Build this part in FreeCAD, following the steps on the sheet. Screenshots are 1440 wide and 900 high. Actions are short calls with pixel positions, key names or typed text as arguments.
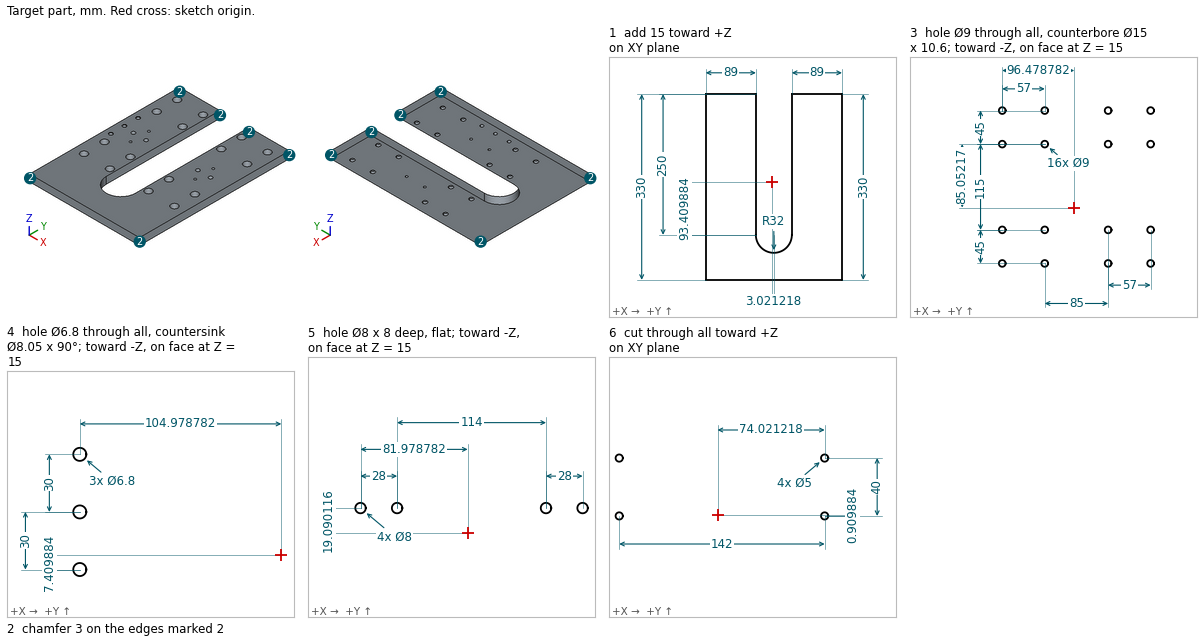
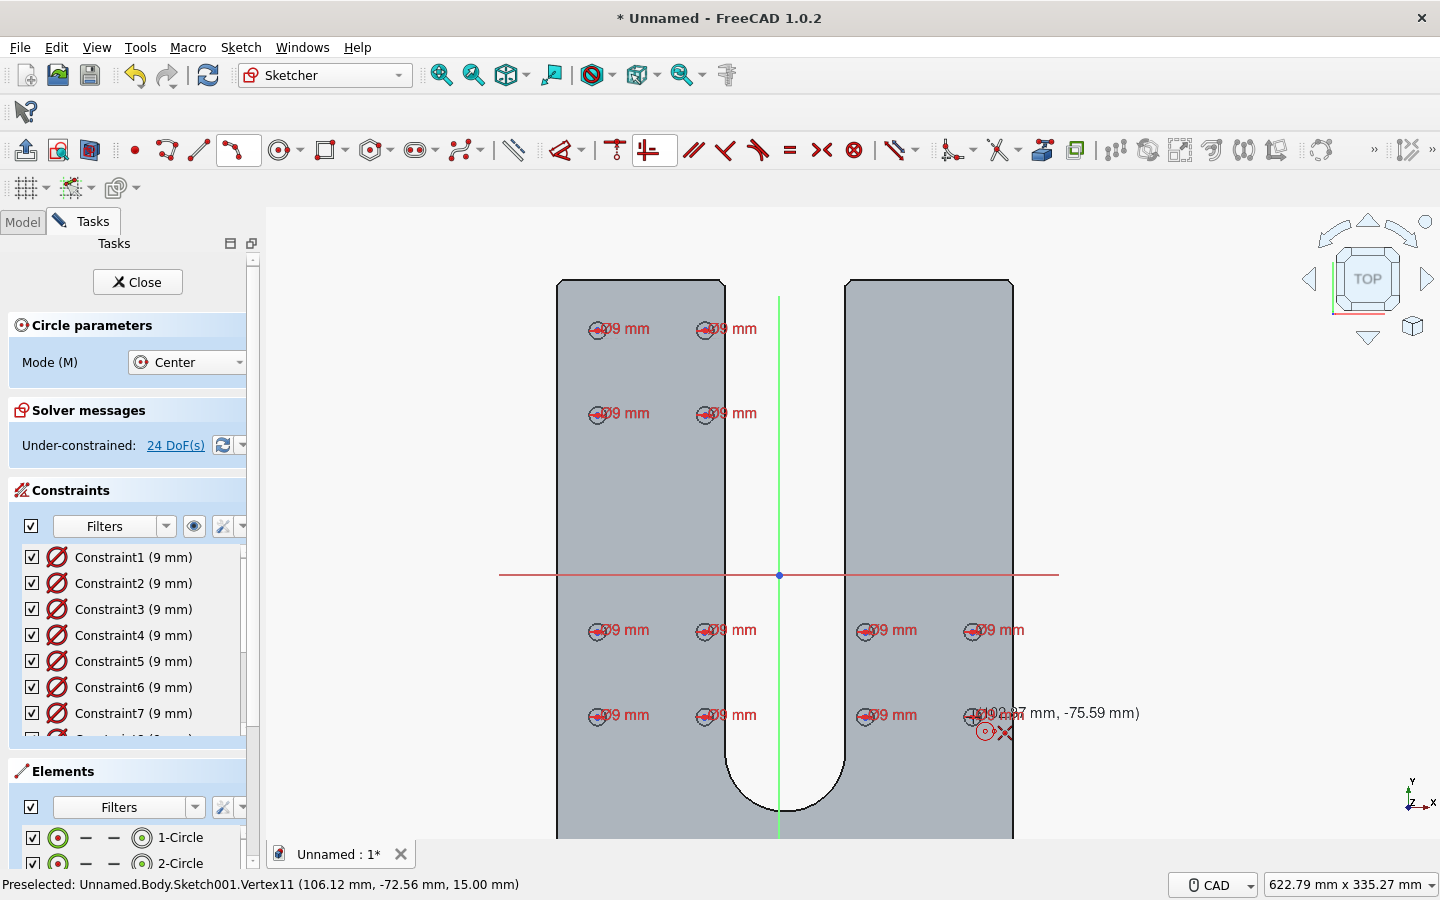
scroll(865, 415, up, 5)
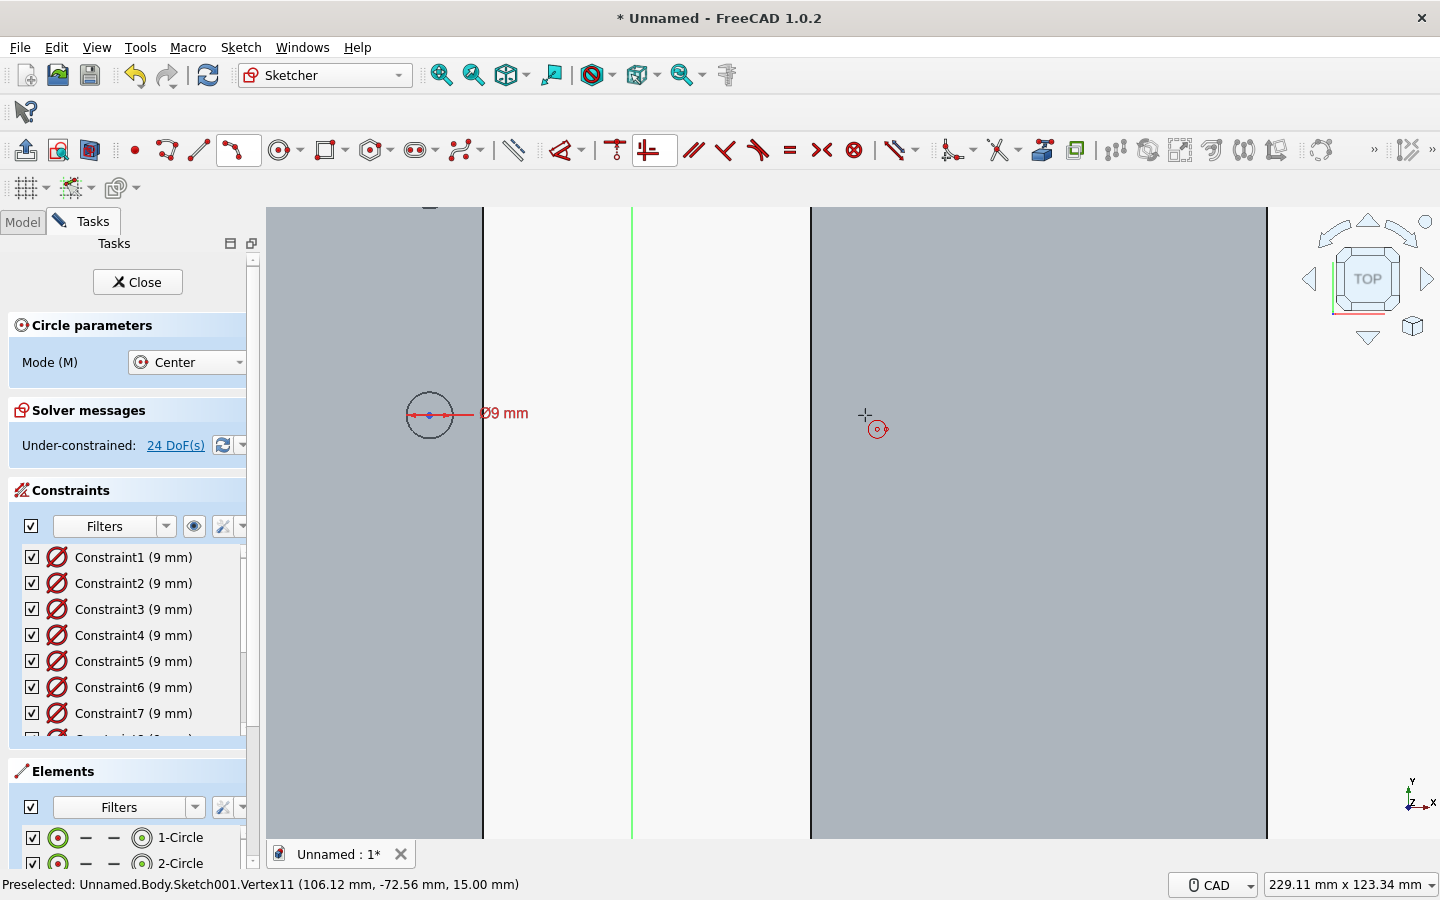
click(865, 415)
move(881, 398)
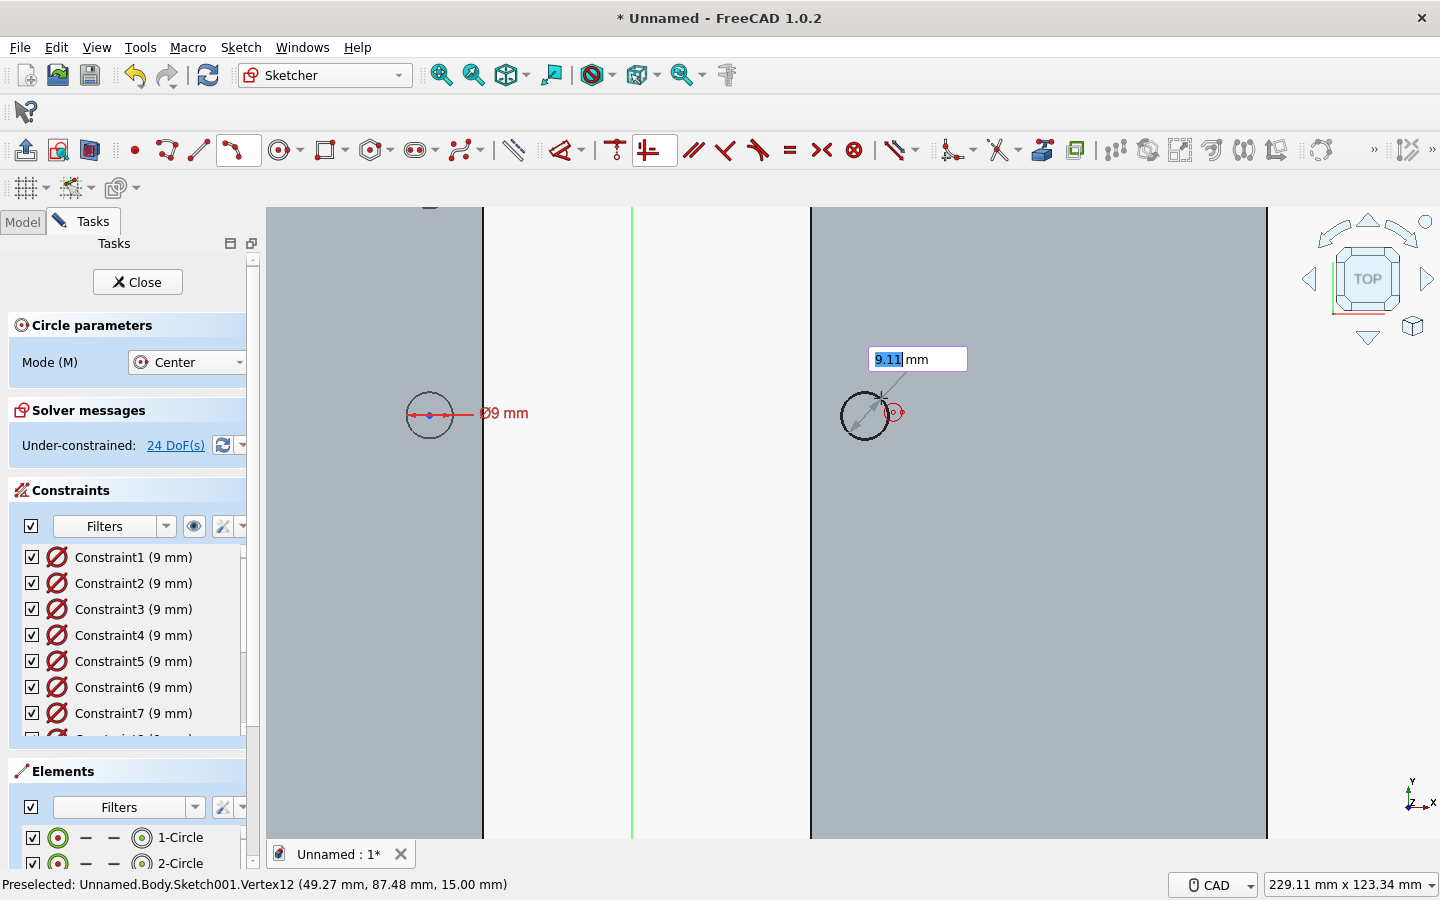
text(9)
key(Return)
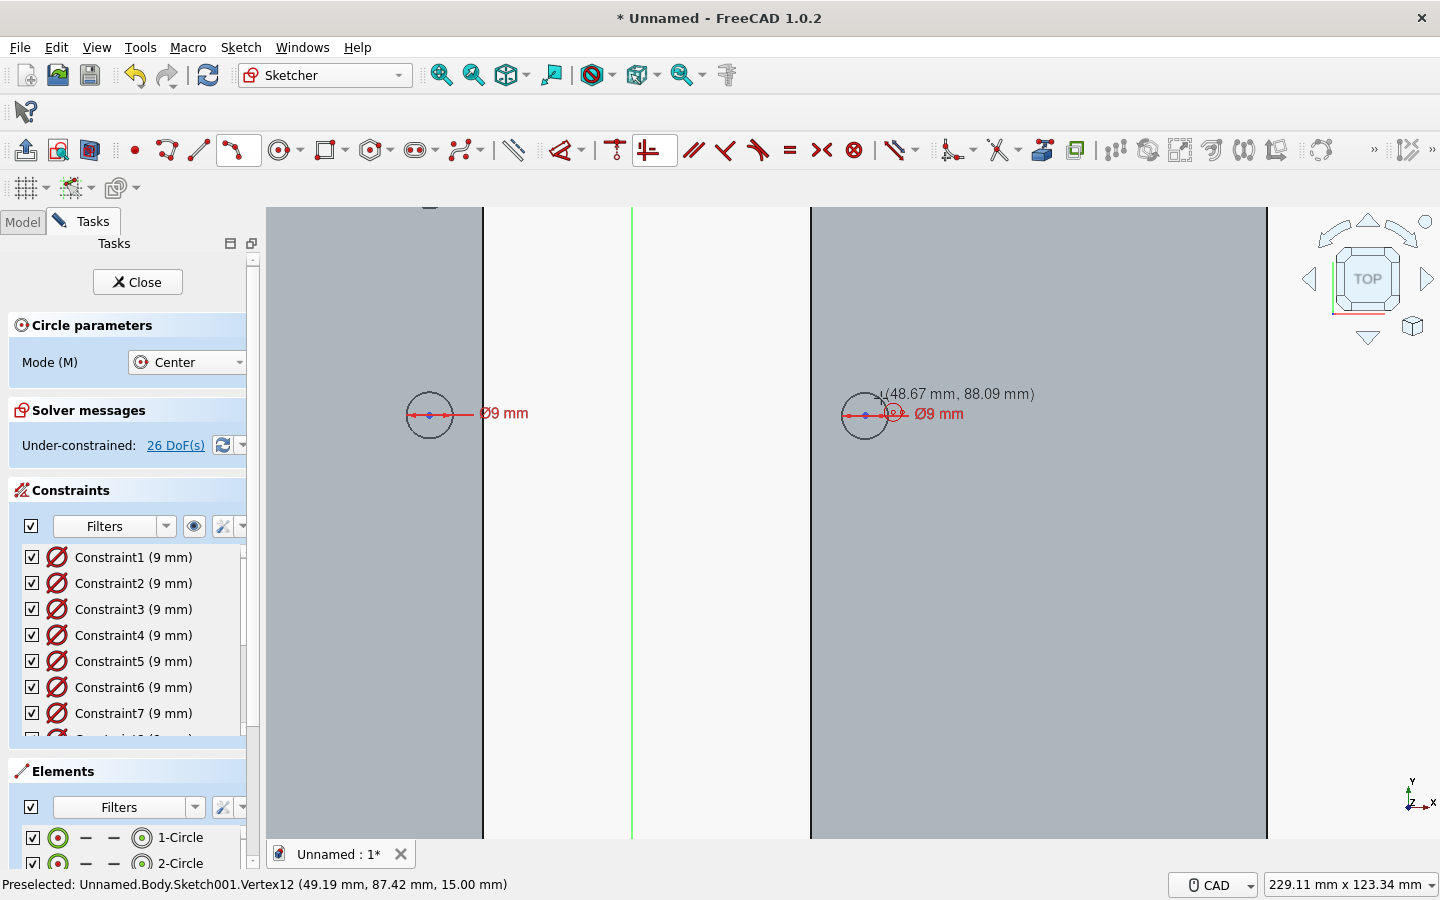
scroll(864, 415, down, 5)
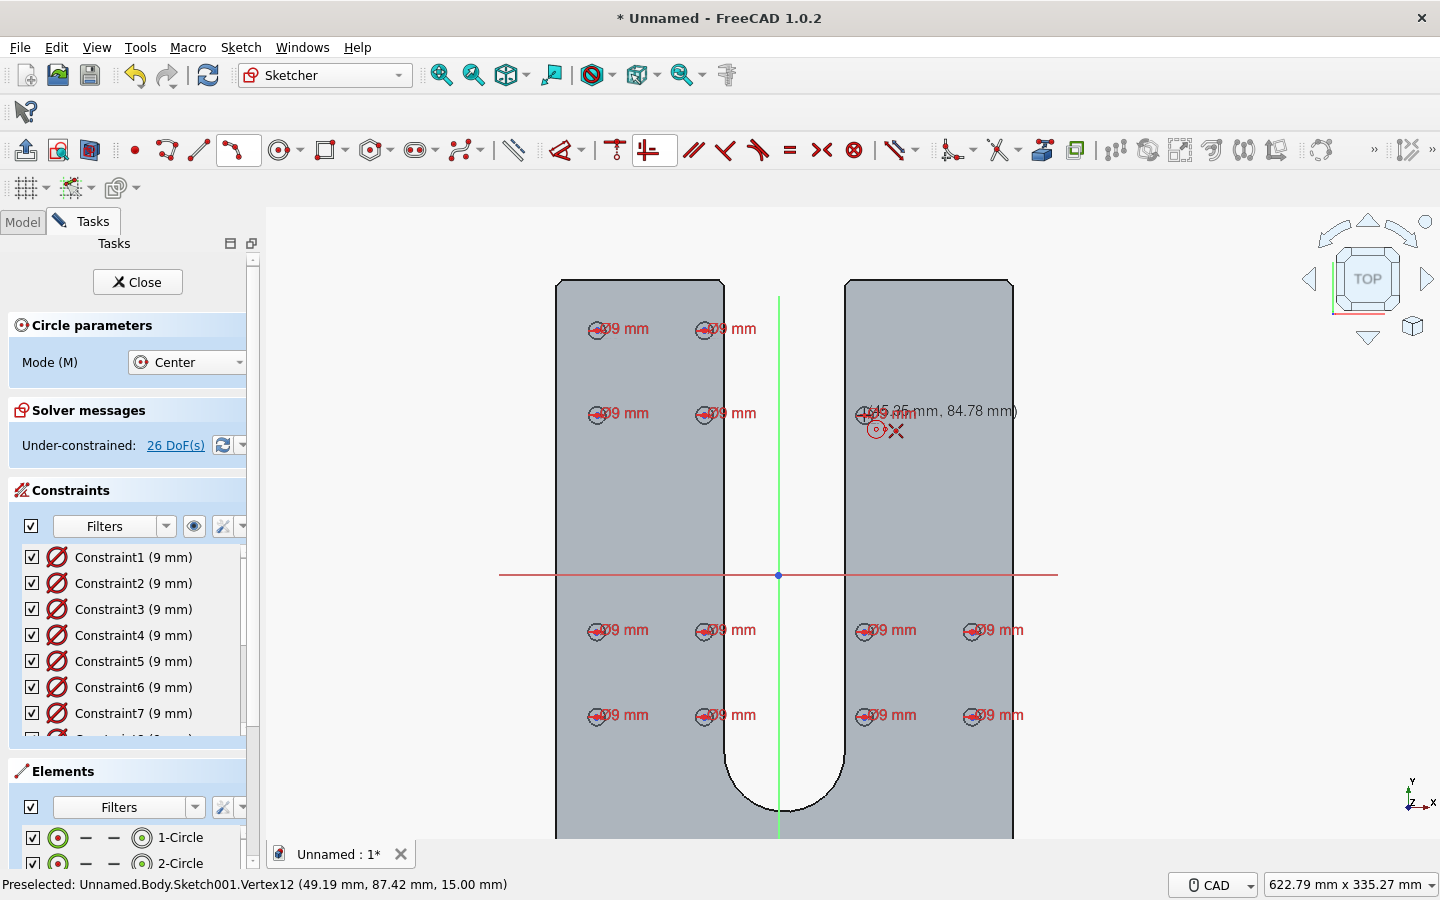
scroll(865, 330, up, 5)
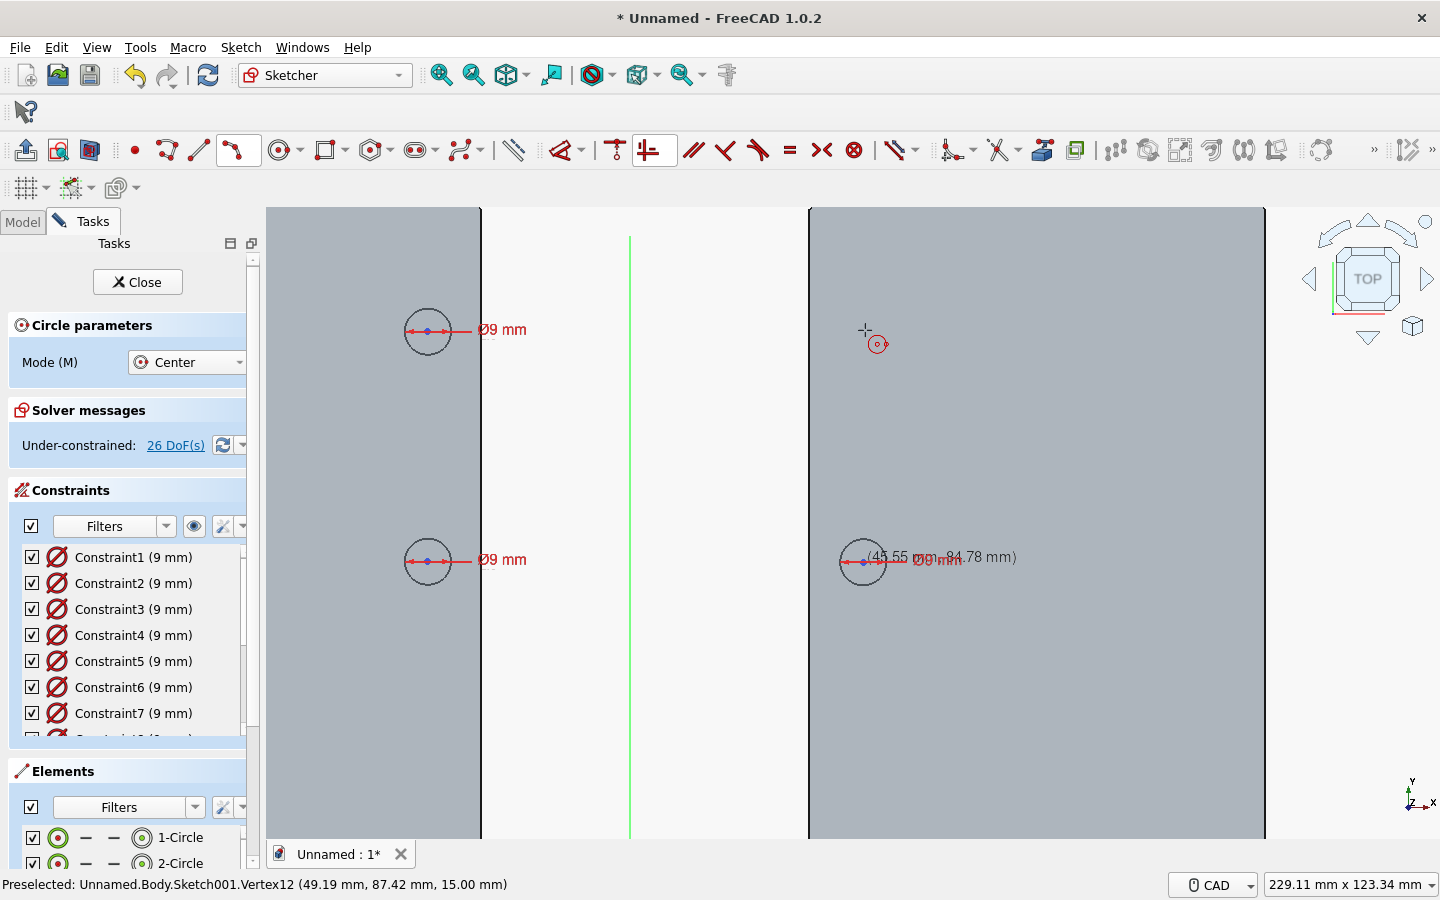
click(863, 330)
move(879, 314)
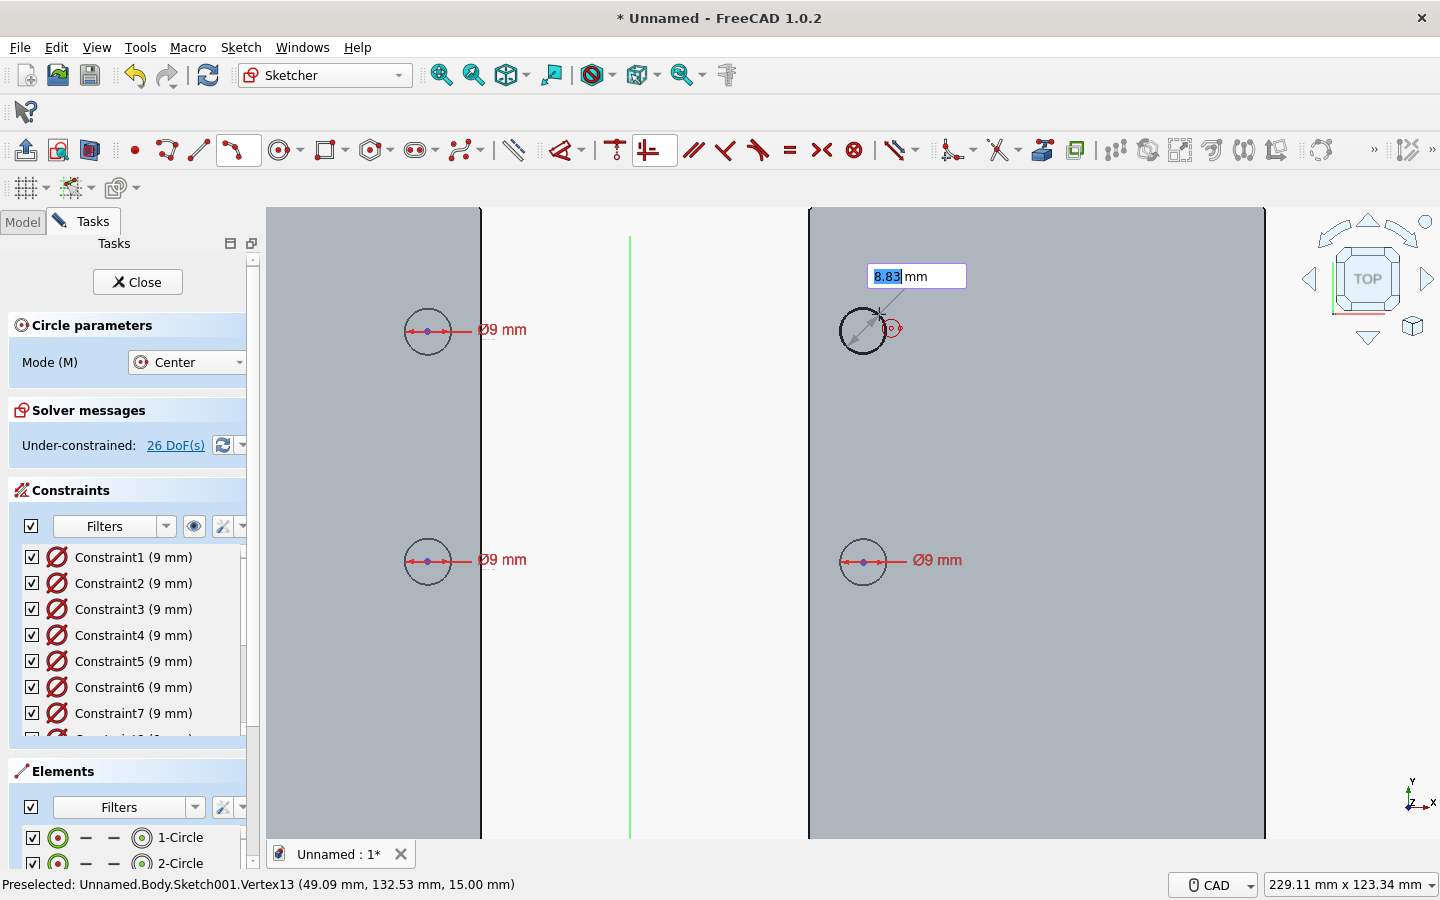
text(9)
key(Return)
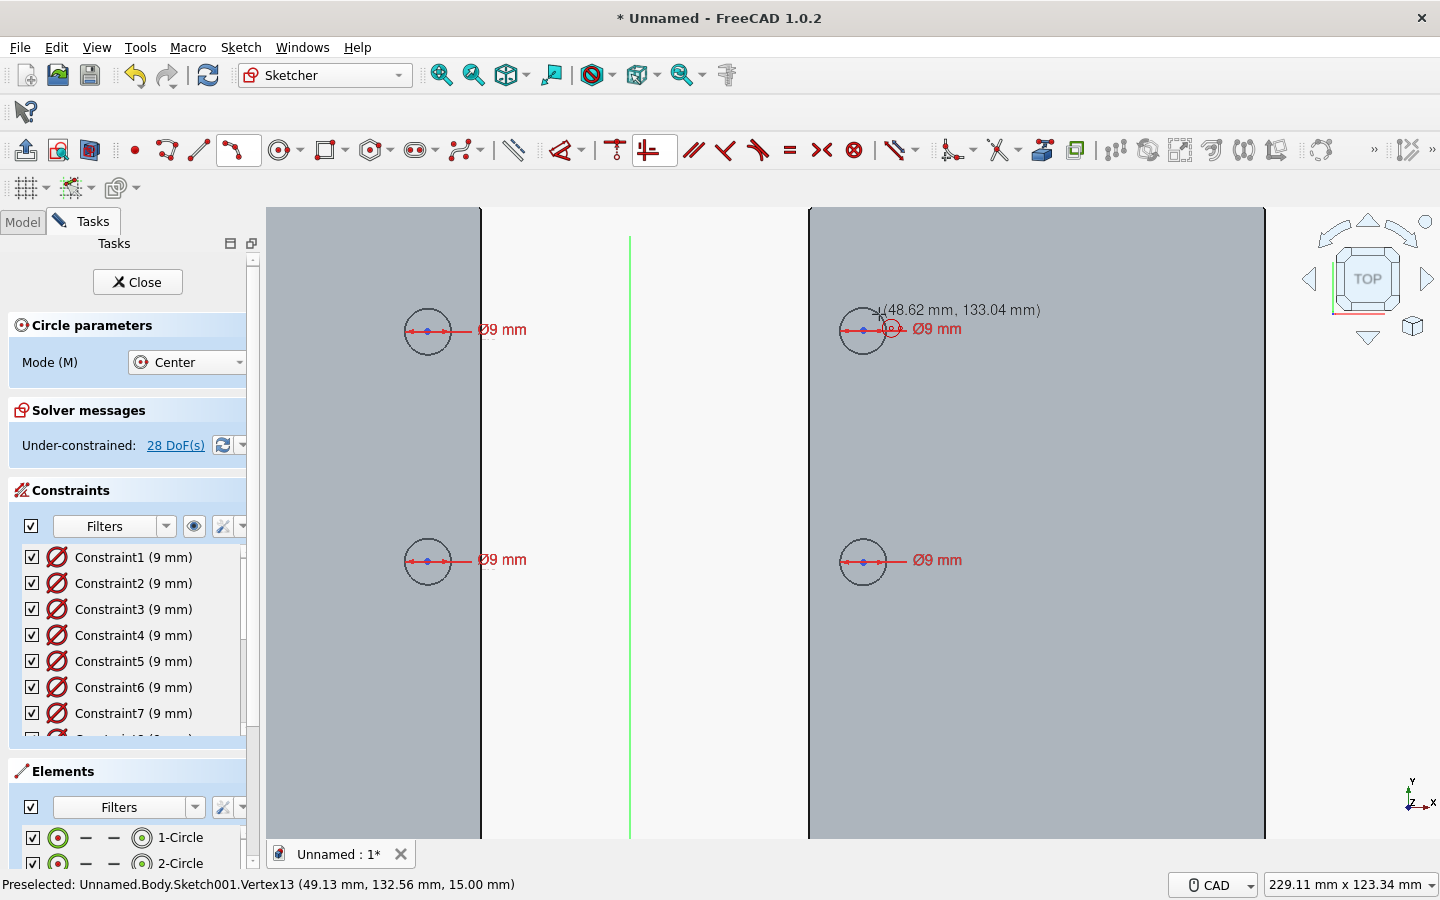
click(1155, 330)
move(1172, 314)